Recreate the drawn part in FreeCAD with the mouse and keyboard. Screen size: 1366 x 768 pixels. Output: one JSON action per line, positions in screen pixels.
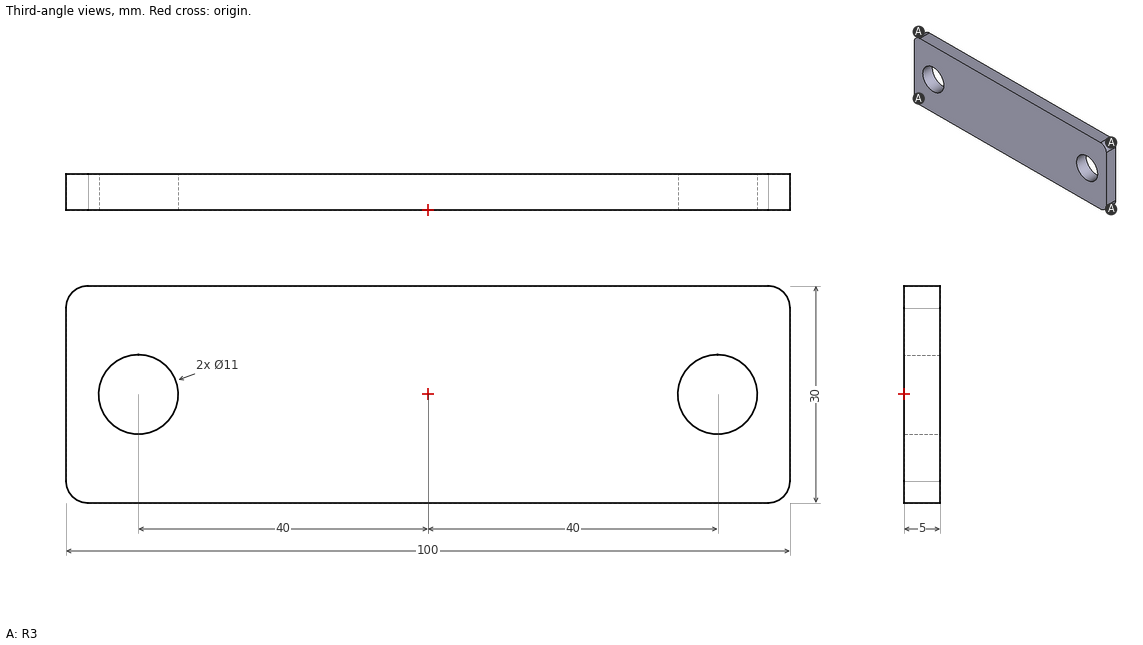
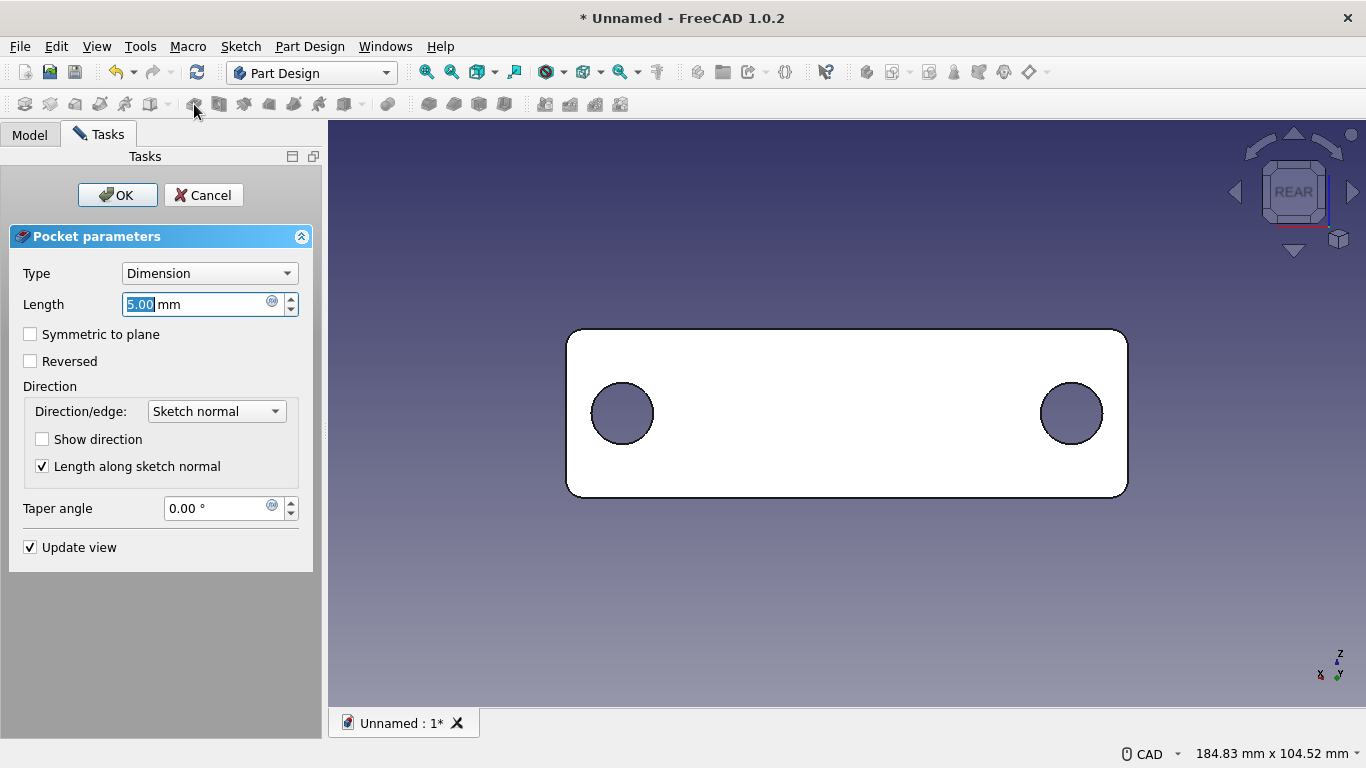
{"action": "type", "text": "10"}
{"action": "key", "text": "Tab"}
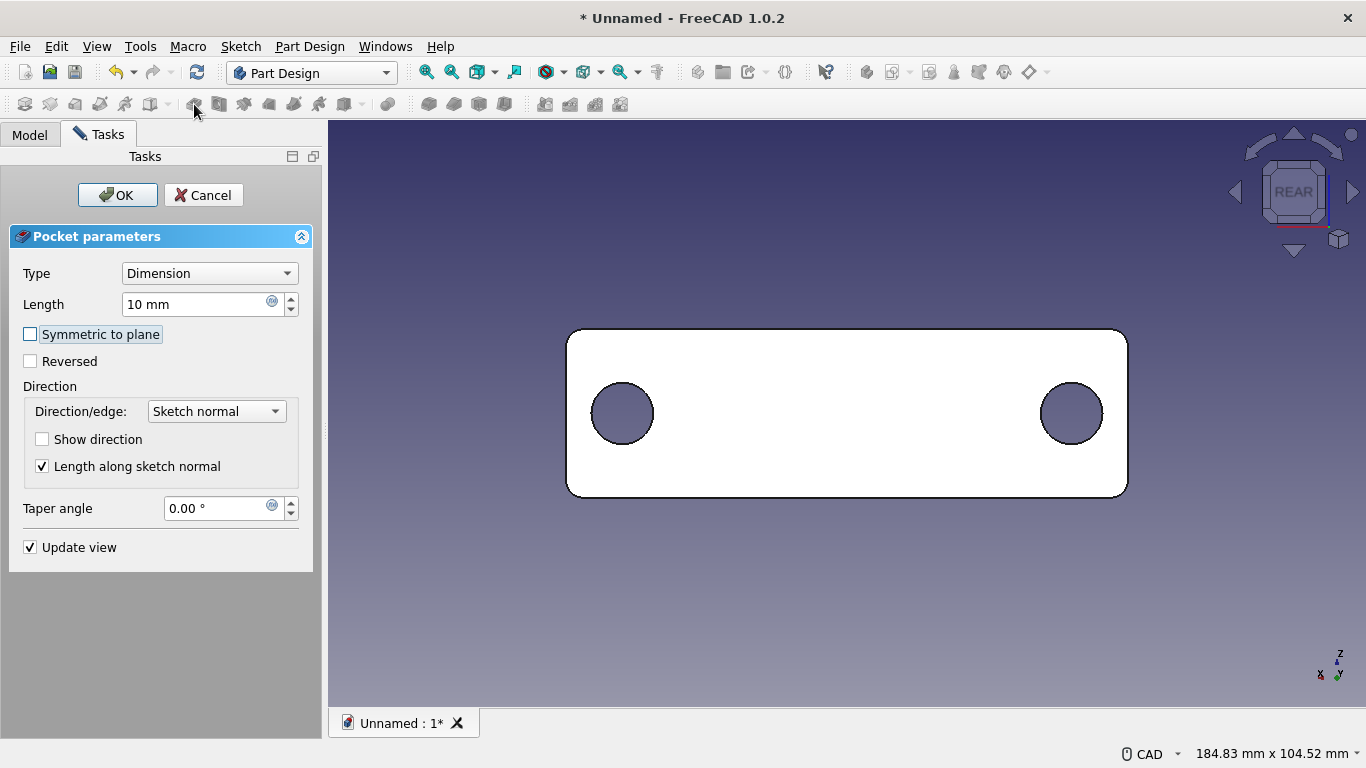
{"action": "left_click", "coordinate": [118, 195]}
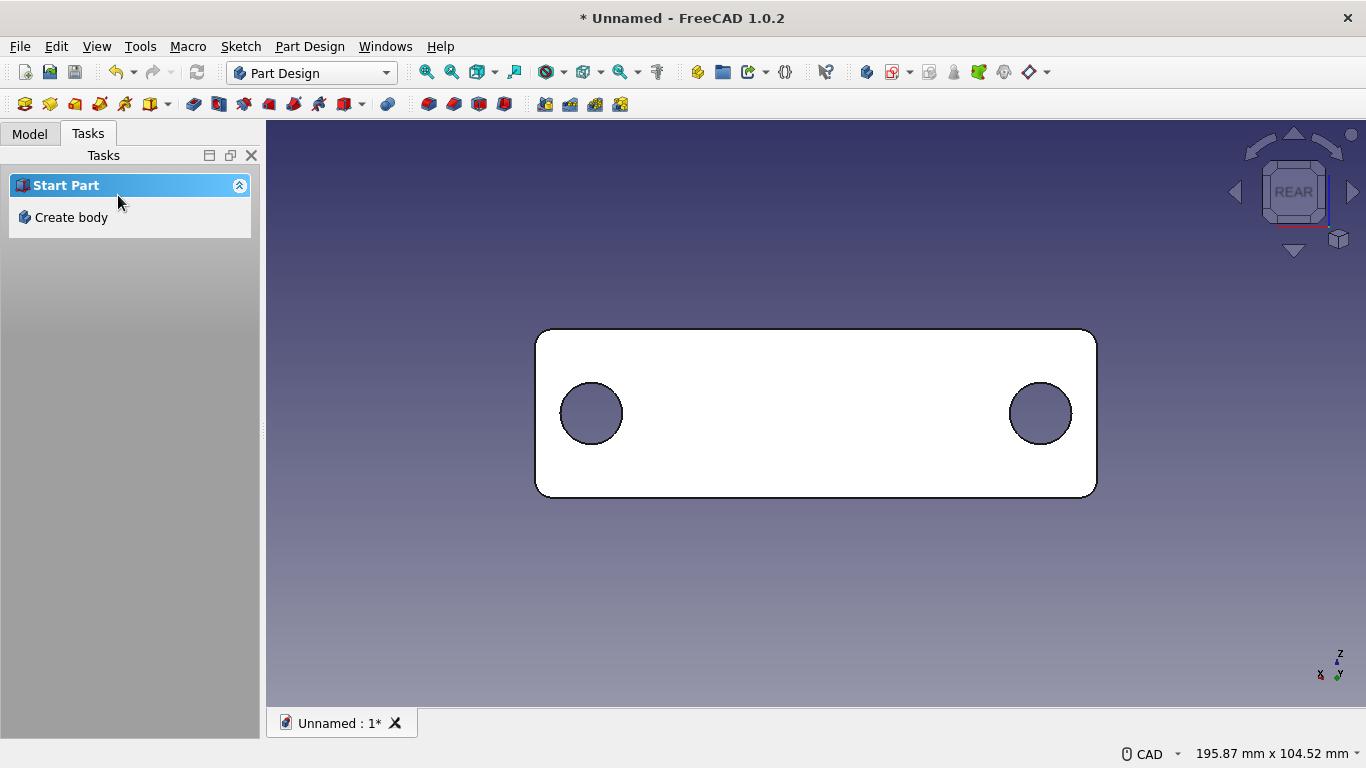
{"action": "key", "text": "0"}